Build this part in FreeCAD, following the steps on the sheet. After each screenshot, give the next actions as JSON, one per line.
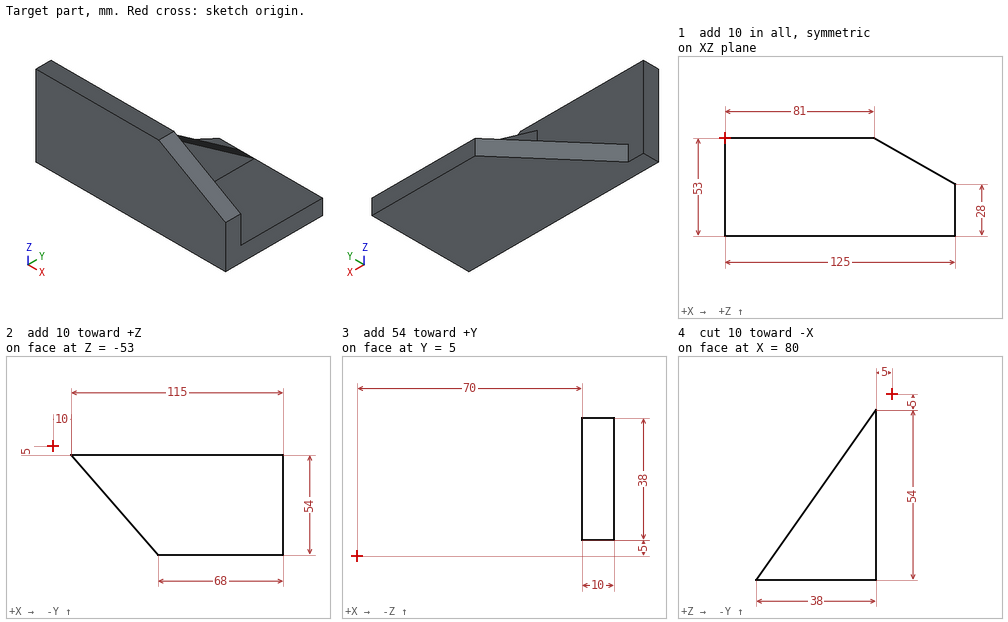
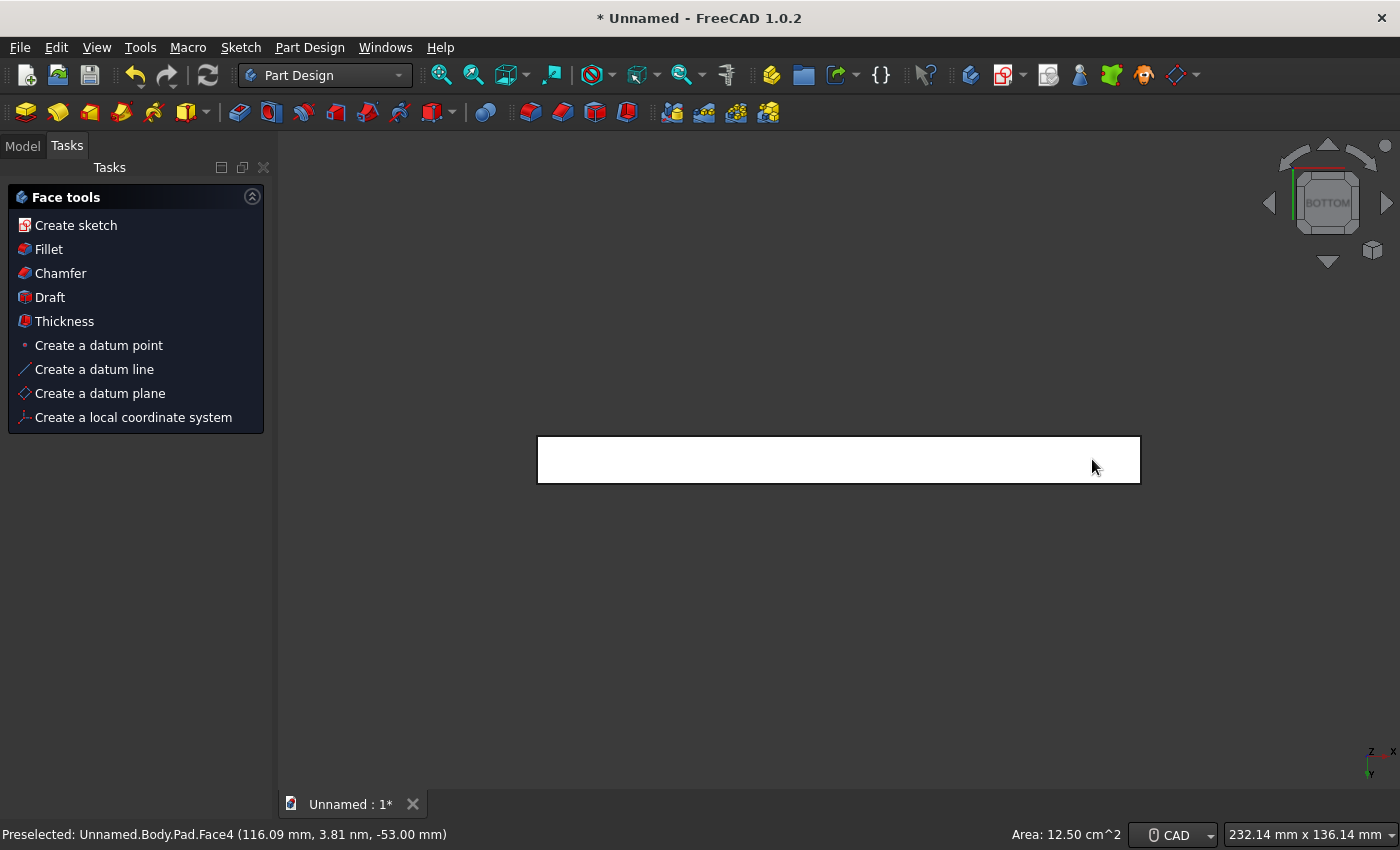
{"action": "left_click", "coordinate": [1004, 76]}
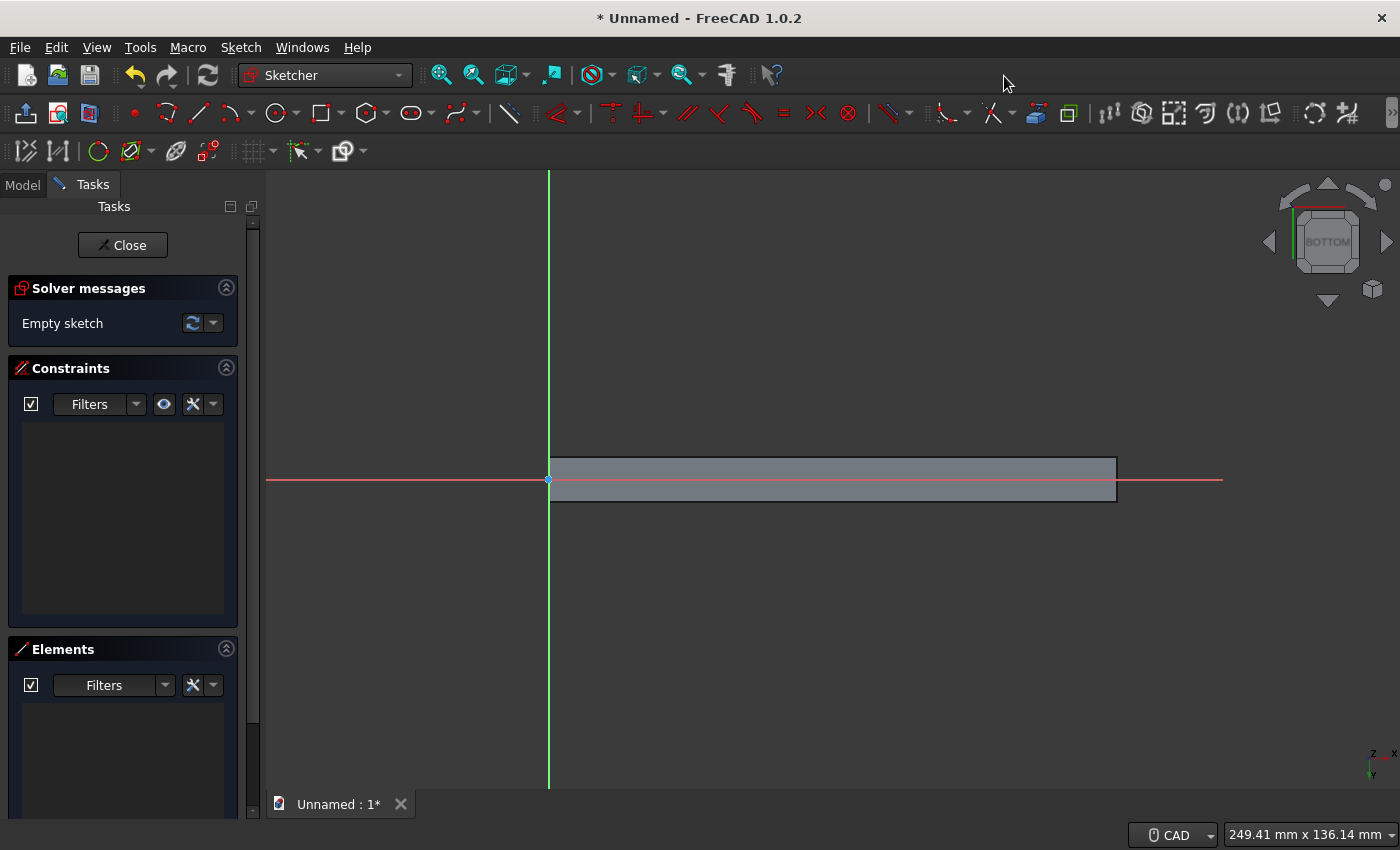
{"action": "scroll", "coordinate": [455, 198], "scroll_direction": "down", "scroll_amount": 1}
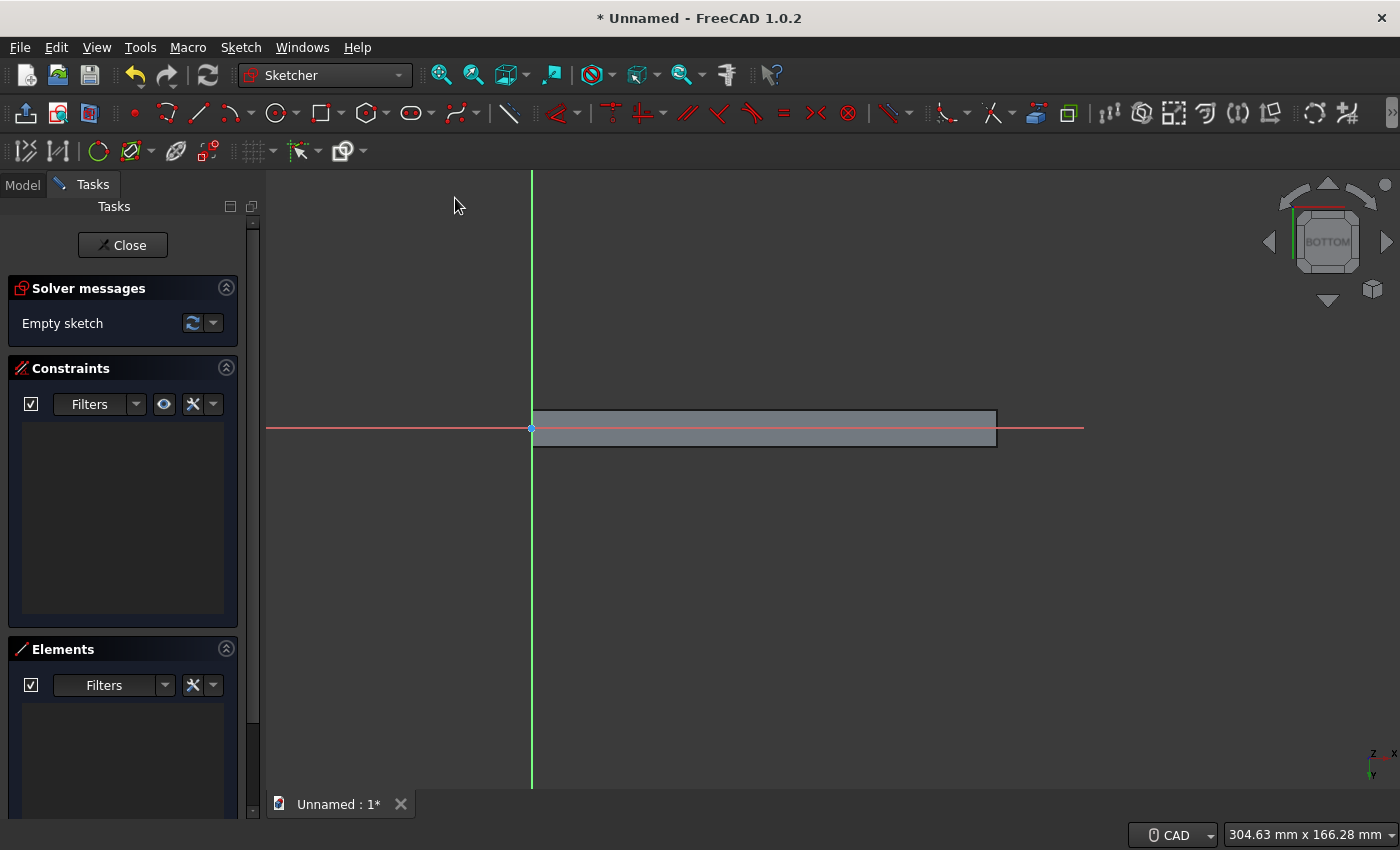
{"action": "scroll", "coordinate": [765, 658], "scroll_direction": "up", "scroll_amount": 2}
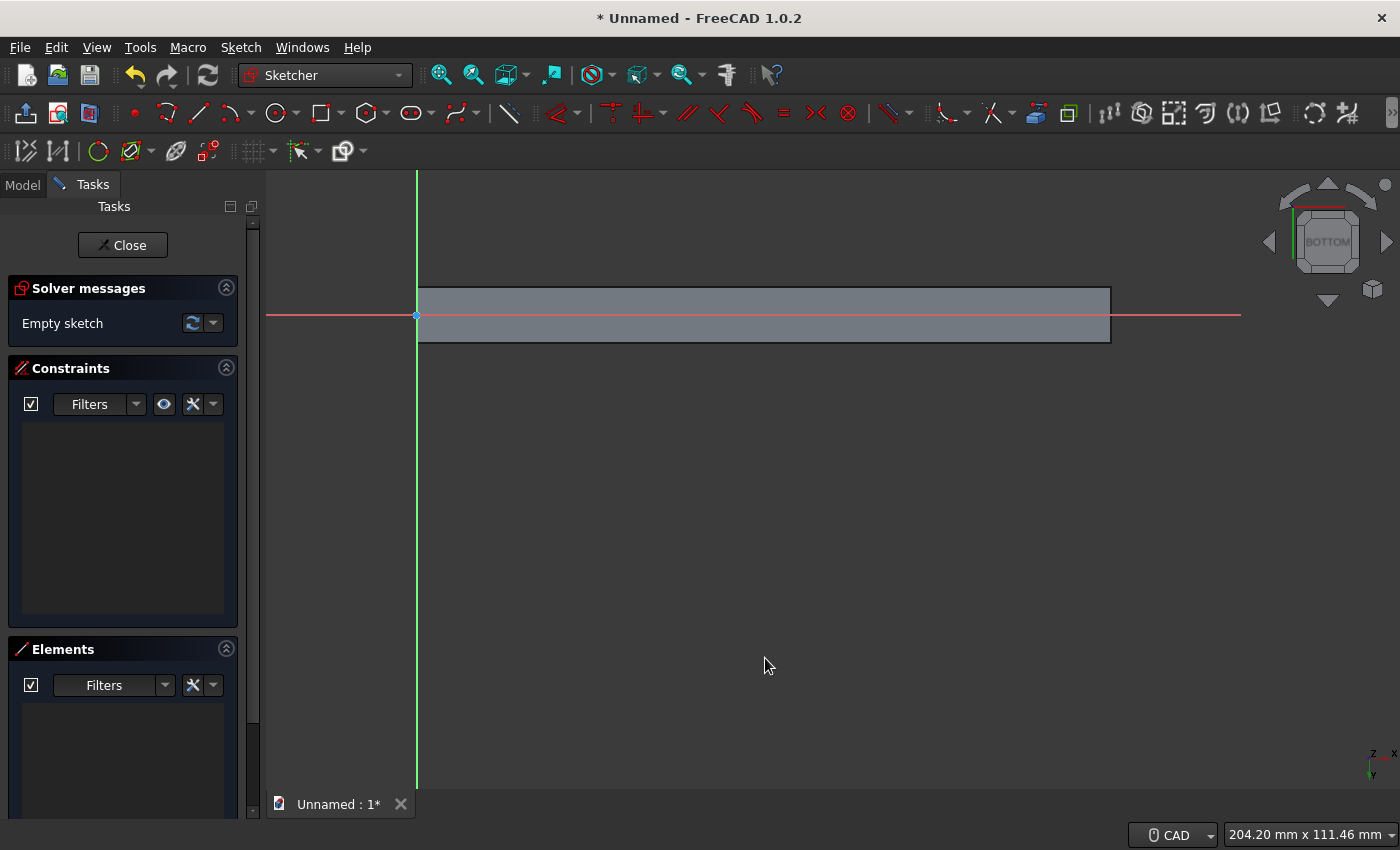
{"action": "left_click", "coordinate": [168, 114]}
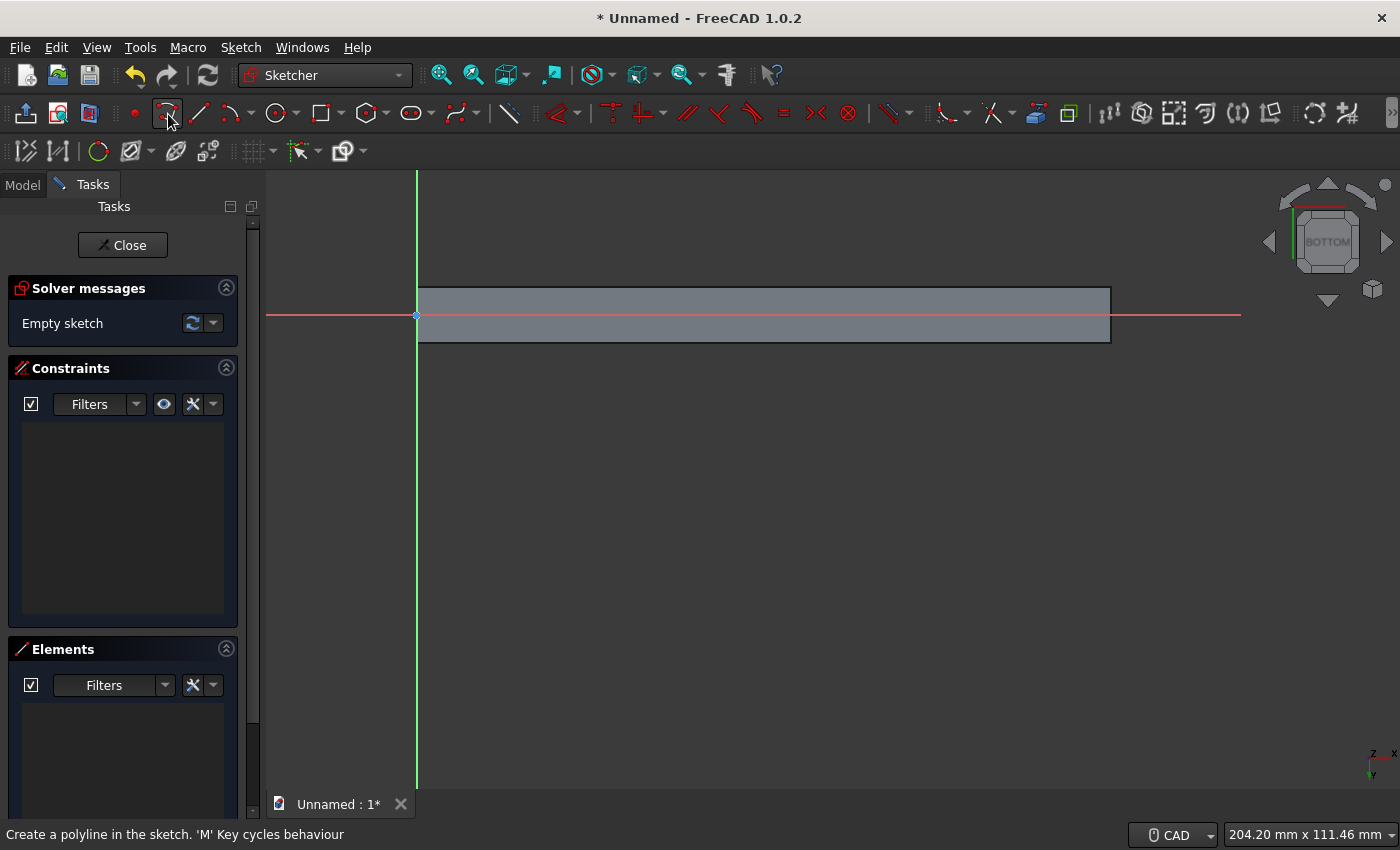
{"action": "left_click", "coordinate": [472, 343]}
{"action": "left_click", "coordinate": [734, 643]}
{"action": "left_click", "coordinate": [1111, 643]}
{"action": "left_click", "coordinate": [1111, 343]}
{"action": "left_click", "coordinate": [472, 344]}
{"action": "key", "text": "Escape"}
{"action": "key", "text": "Escape"}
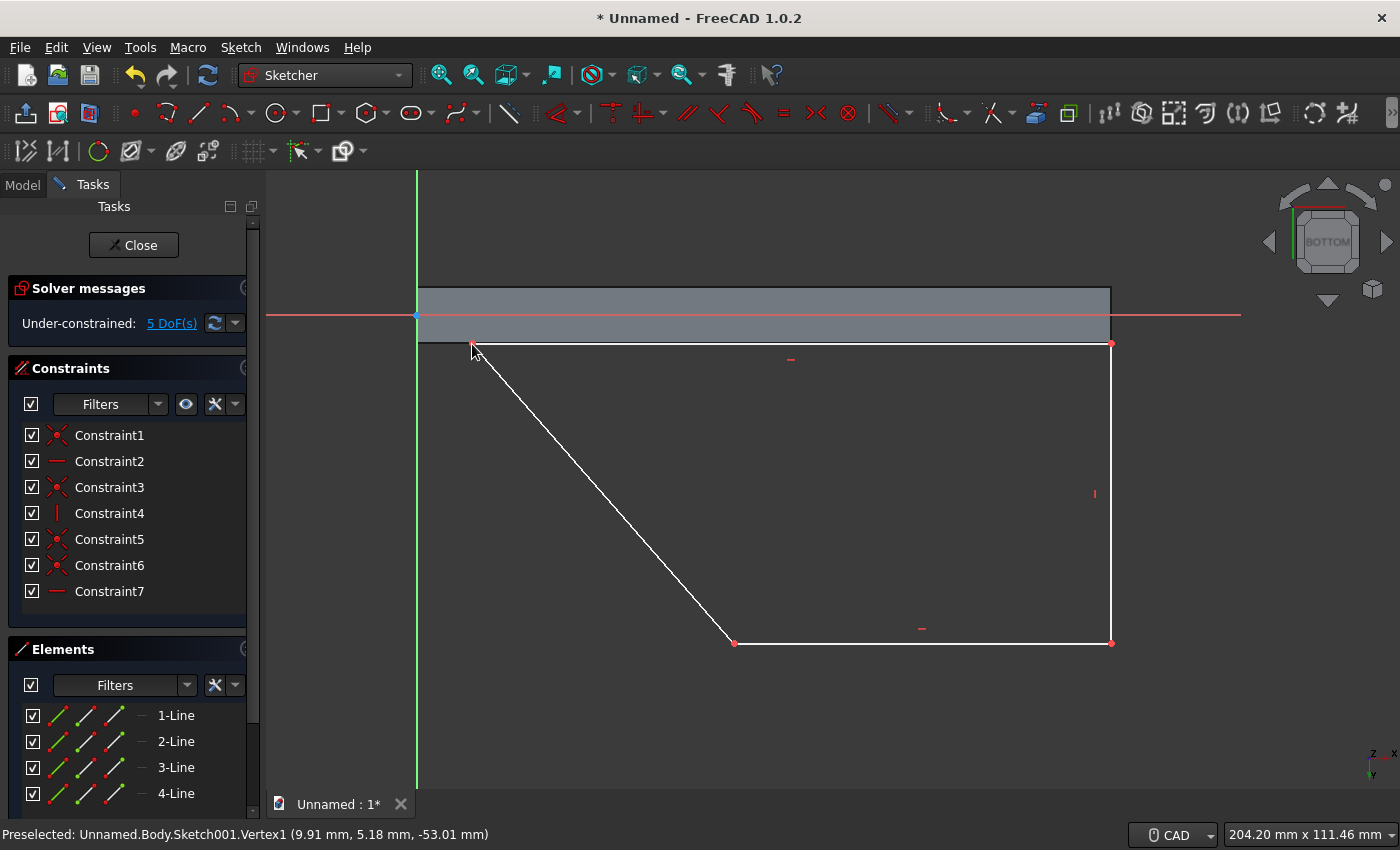
{"action": "key", "text": "d"}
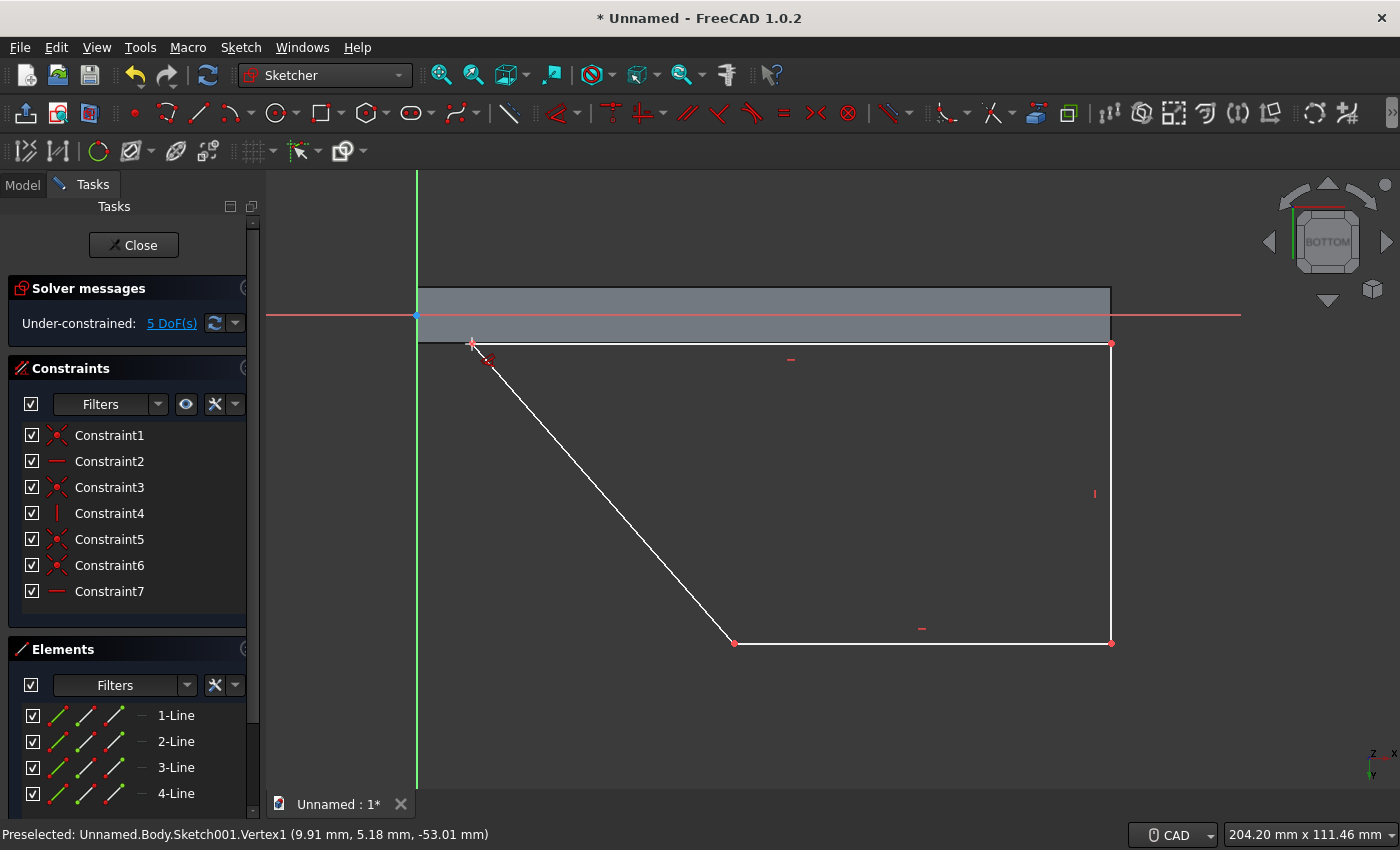
{"action": "left_click", "coordinate": [847, 644]}
{"action": "left_click", "coordinate": [923, 678]}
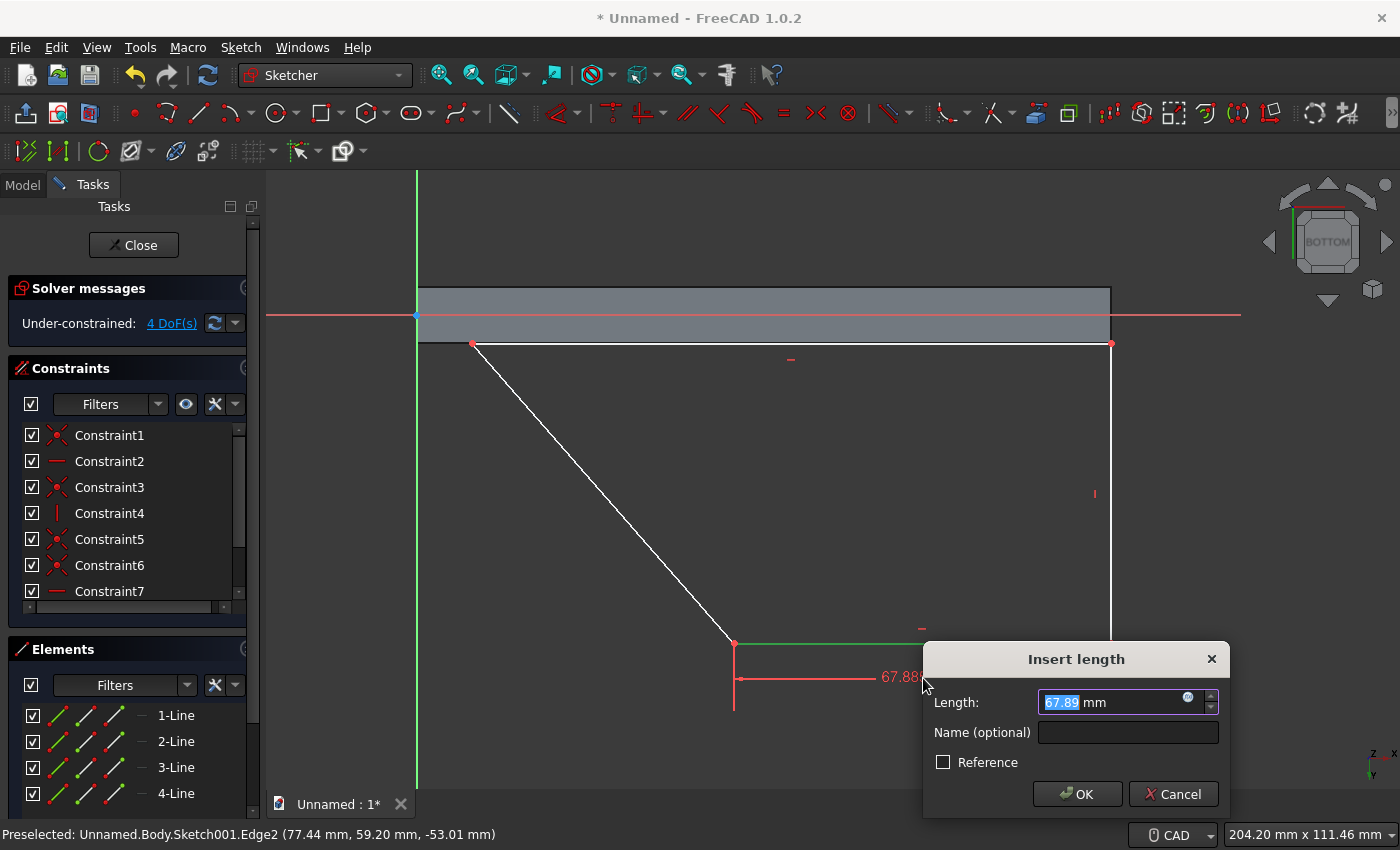
{"action": "type", "text": "68"}
{"action": "key", "text": "Return"}